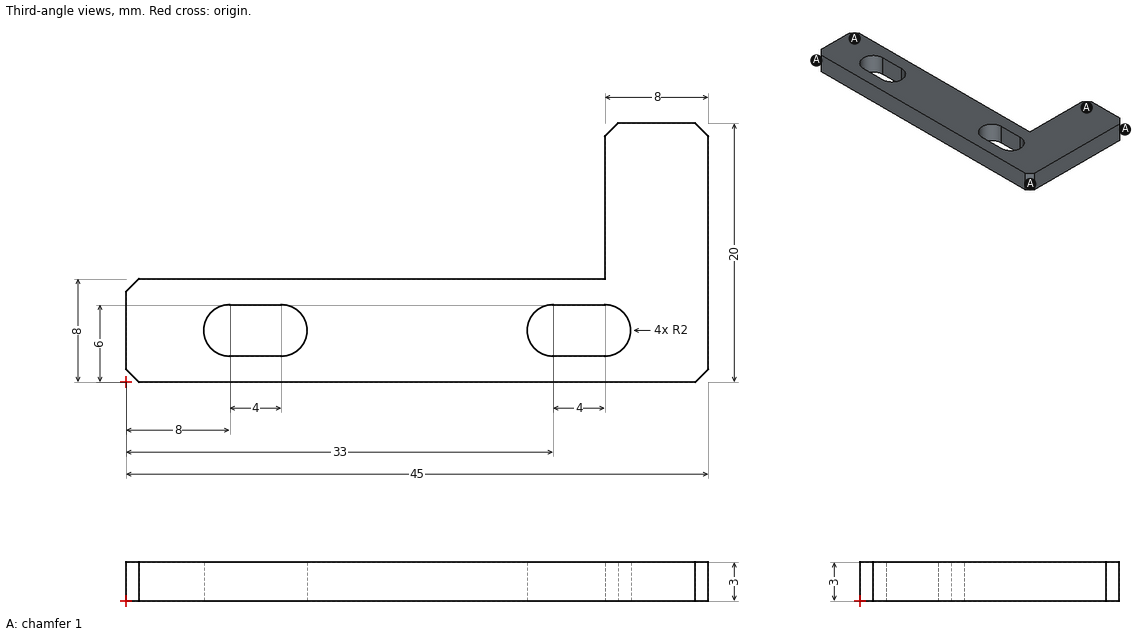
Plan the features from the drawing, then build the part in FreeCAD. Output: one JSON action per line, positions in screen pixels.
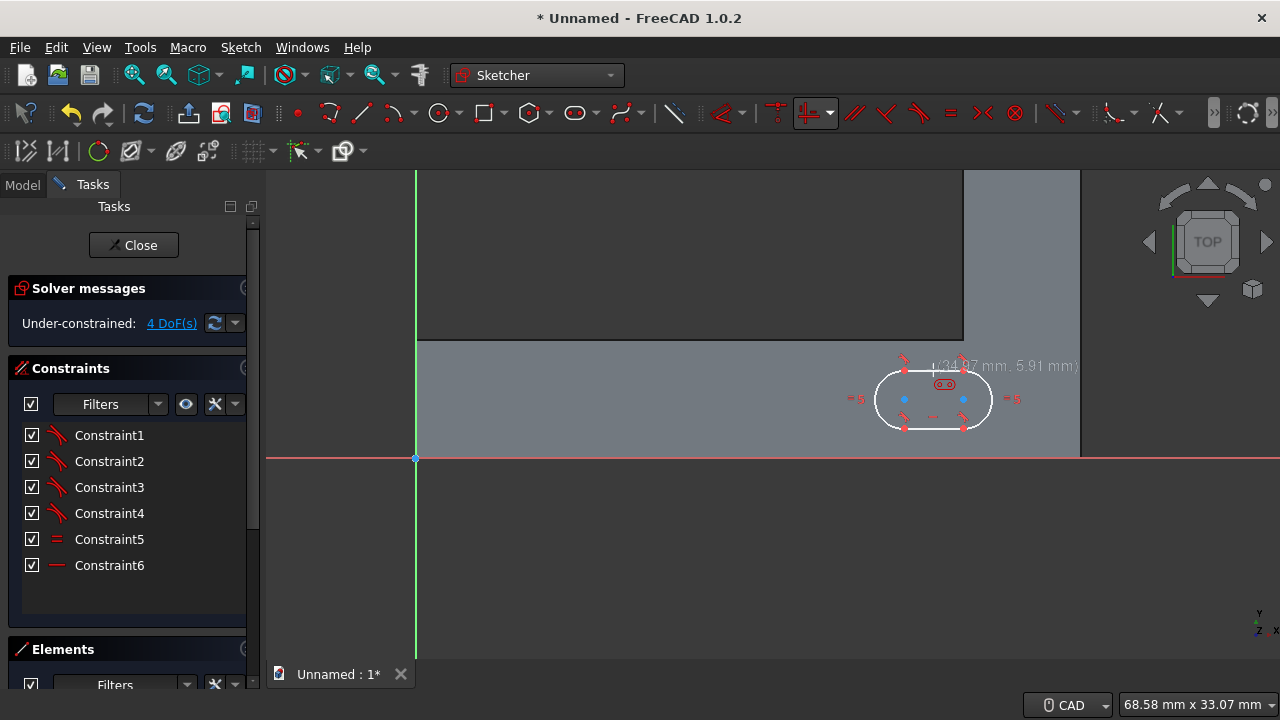
{"action": "left_click", "coordinate": [534, 399]}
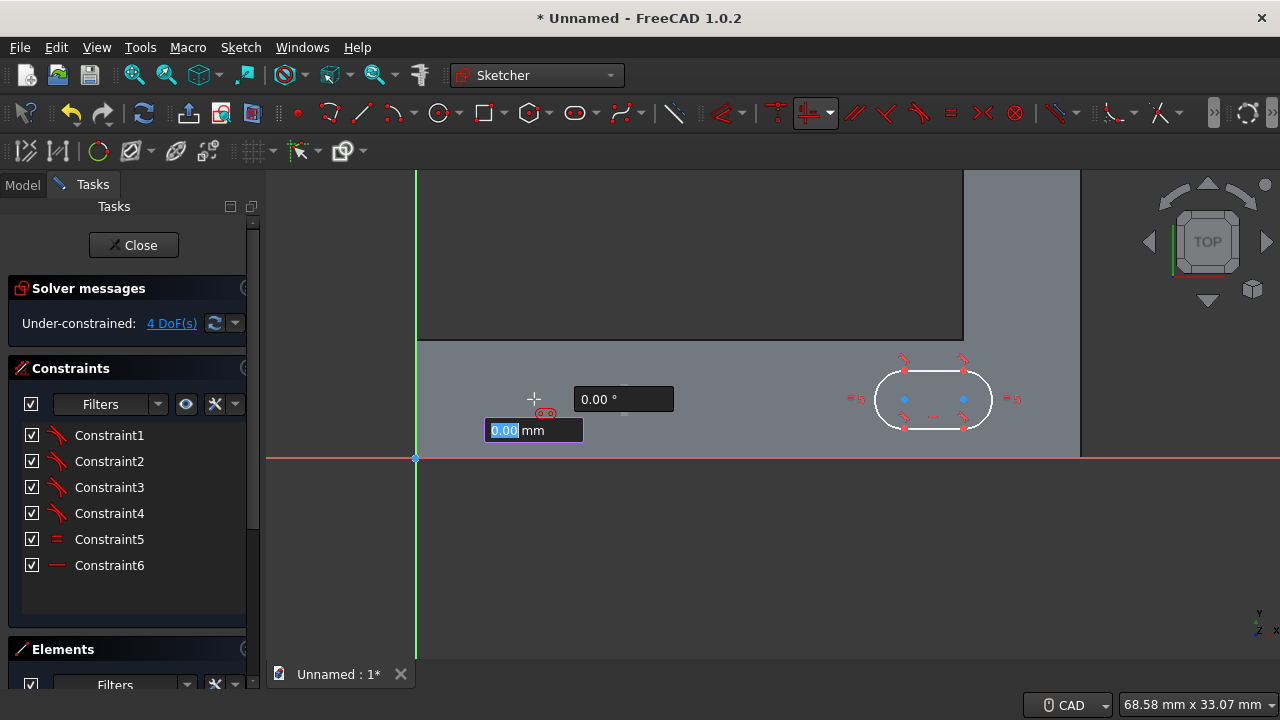
{"action": "left_click", "coordinate": [593, 399]}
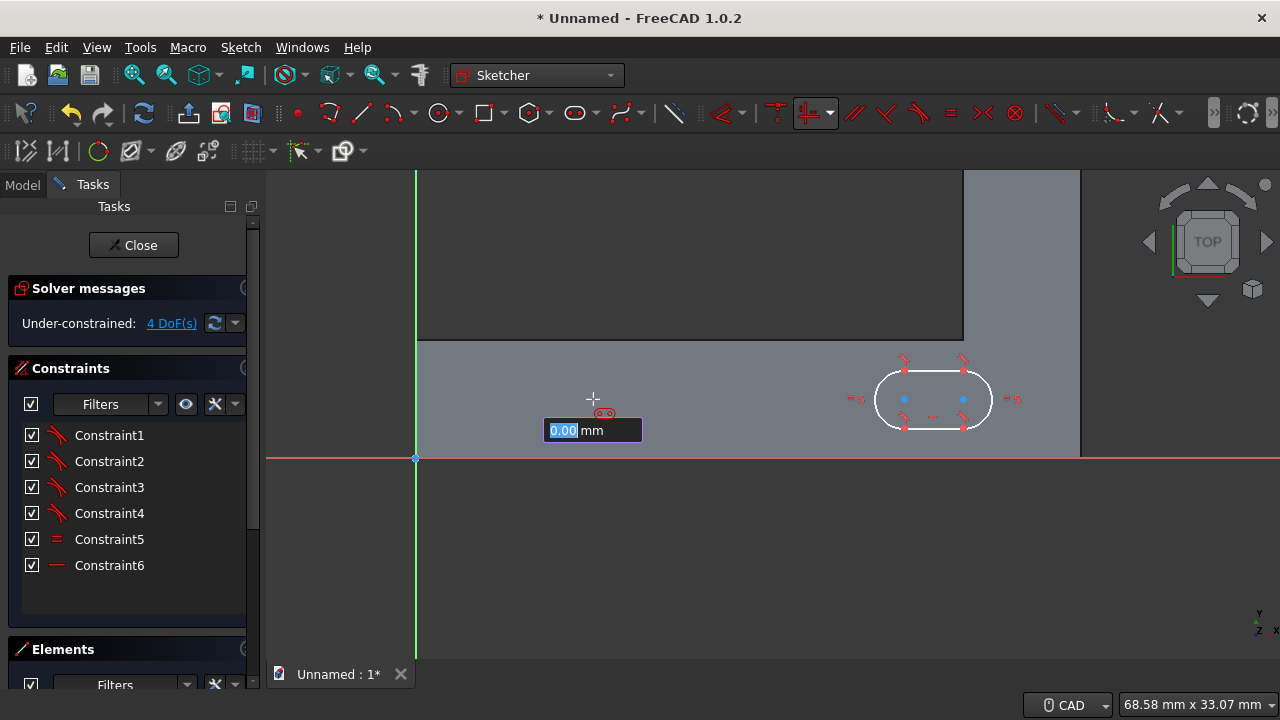
{"action": "left_click", "coordinate": [564, 370]}
{"action": "key", "text": "Escape"}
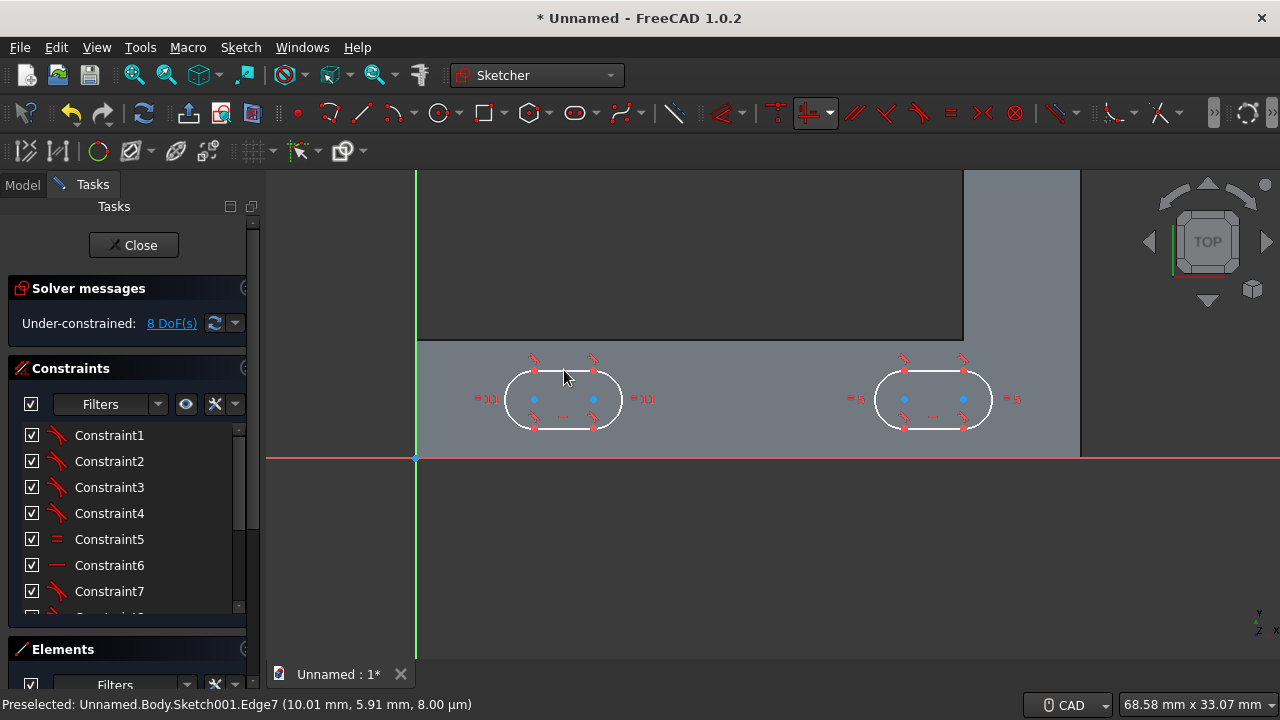
{"action": "left_click", "coordinate": [881, 383]}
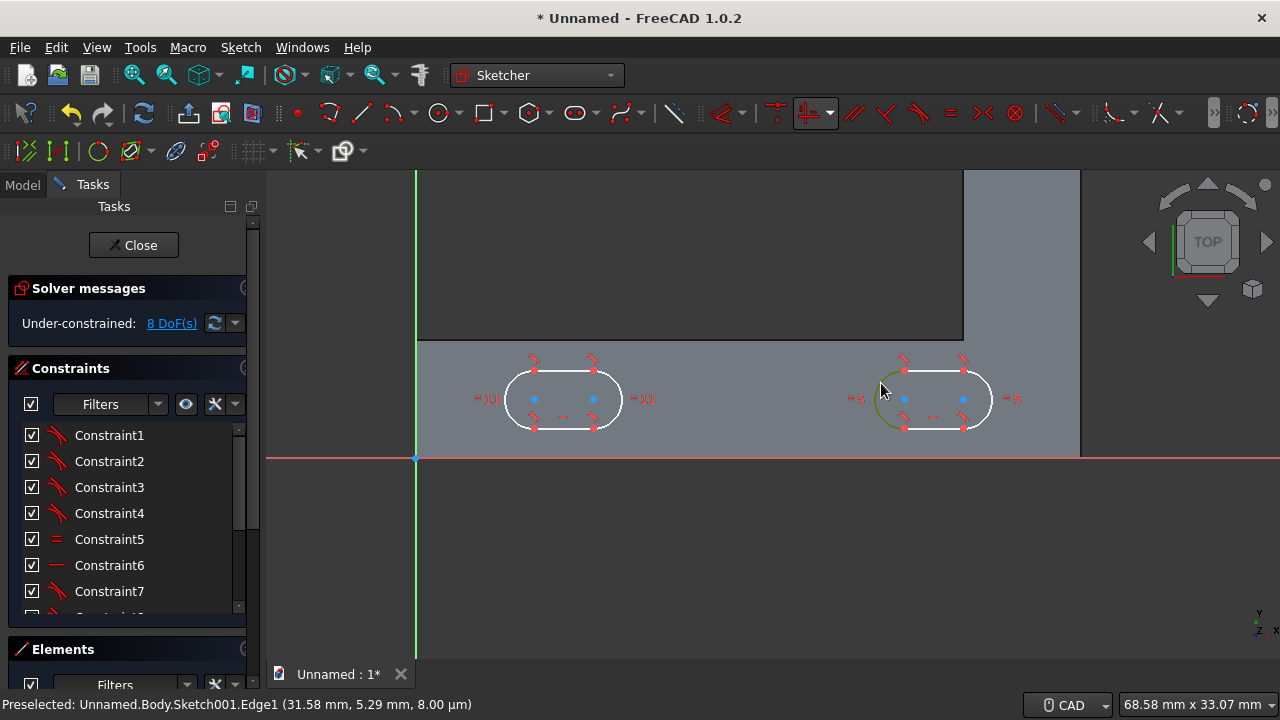
{"action": "left_click", "coordinate": [511, 383]}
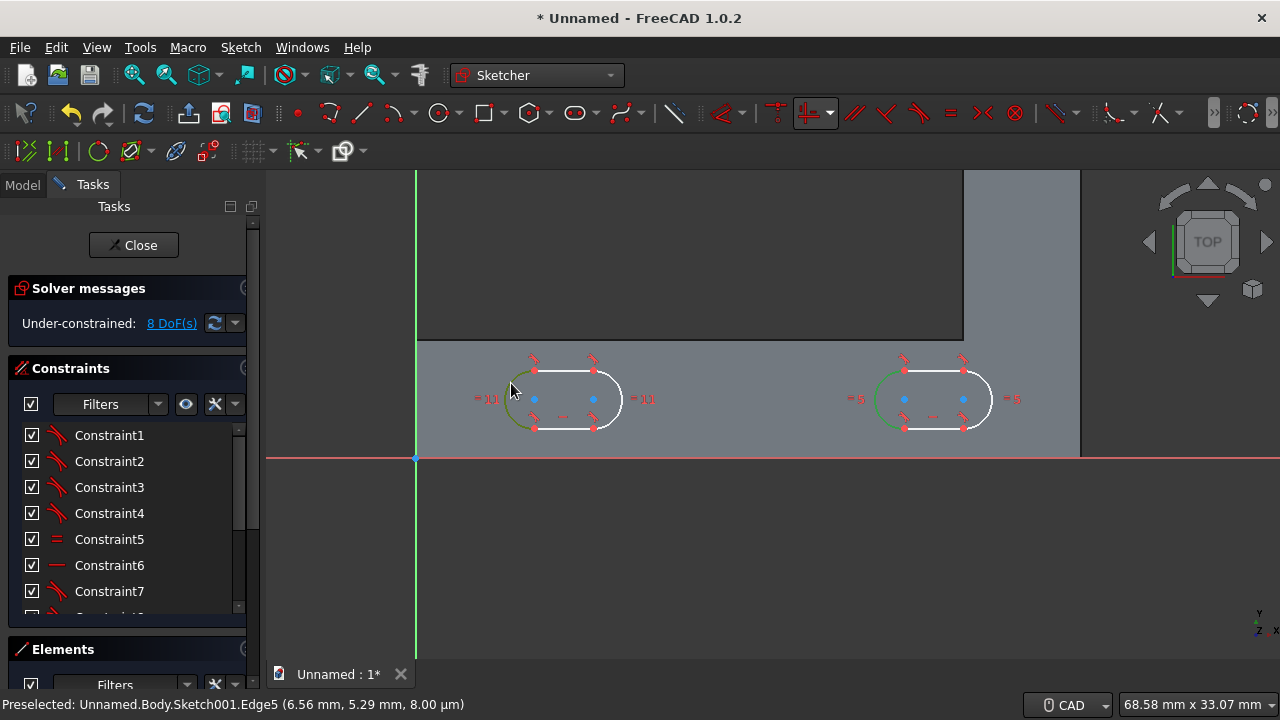
{"action": "left_click", "coordinate": [952, 114]}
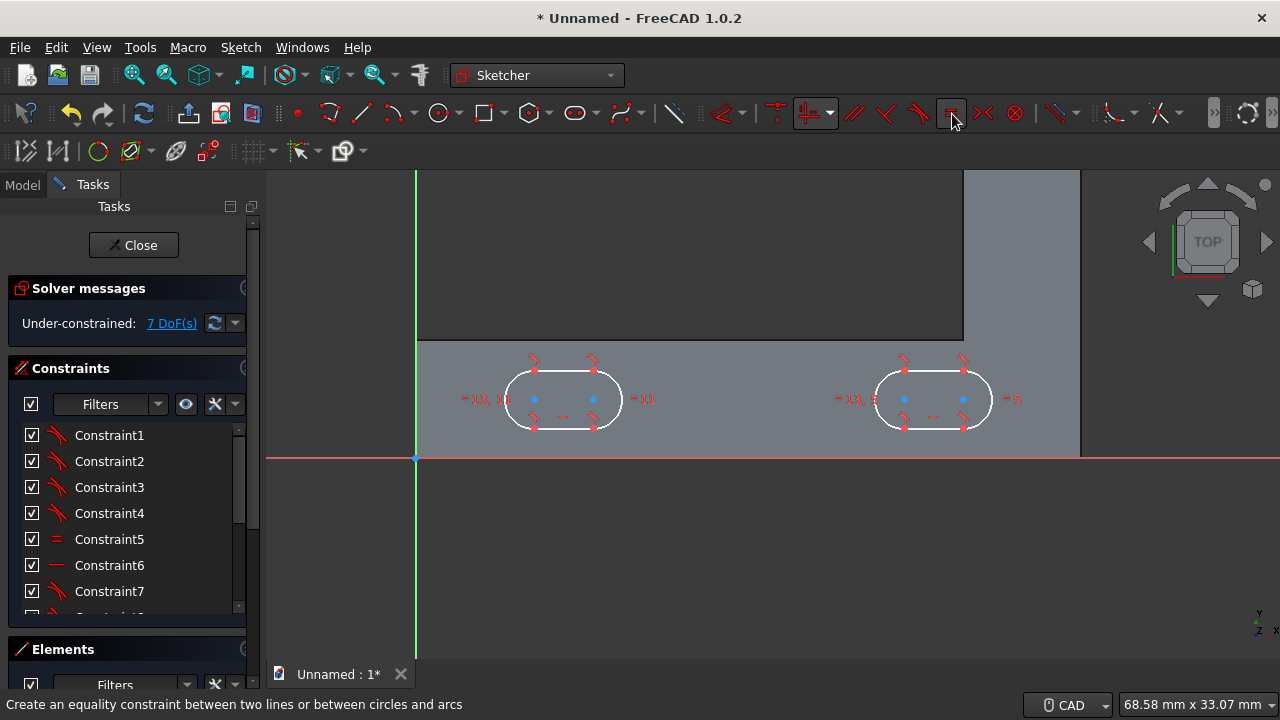
{"action": "left_click", "coordinate": [722, 114]}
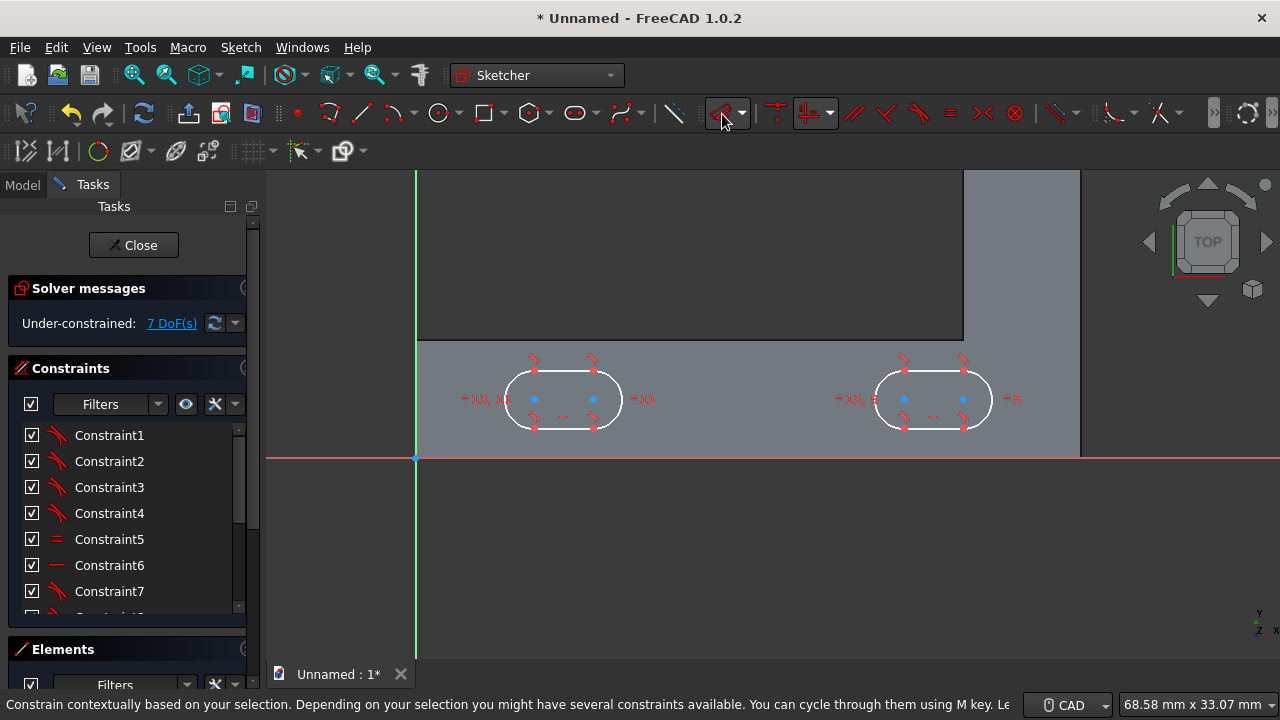
{"action": "scroll", "coordinate": [881, 383], "scroll_direction": "up", "scroll_amount": 2}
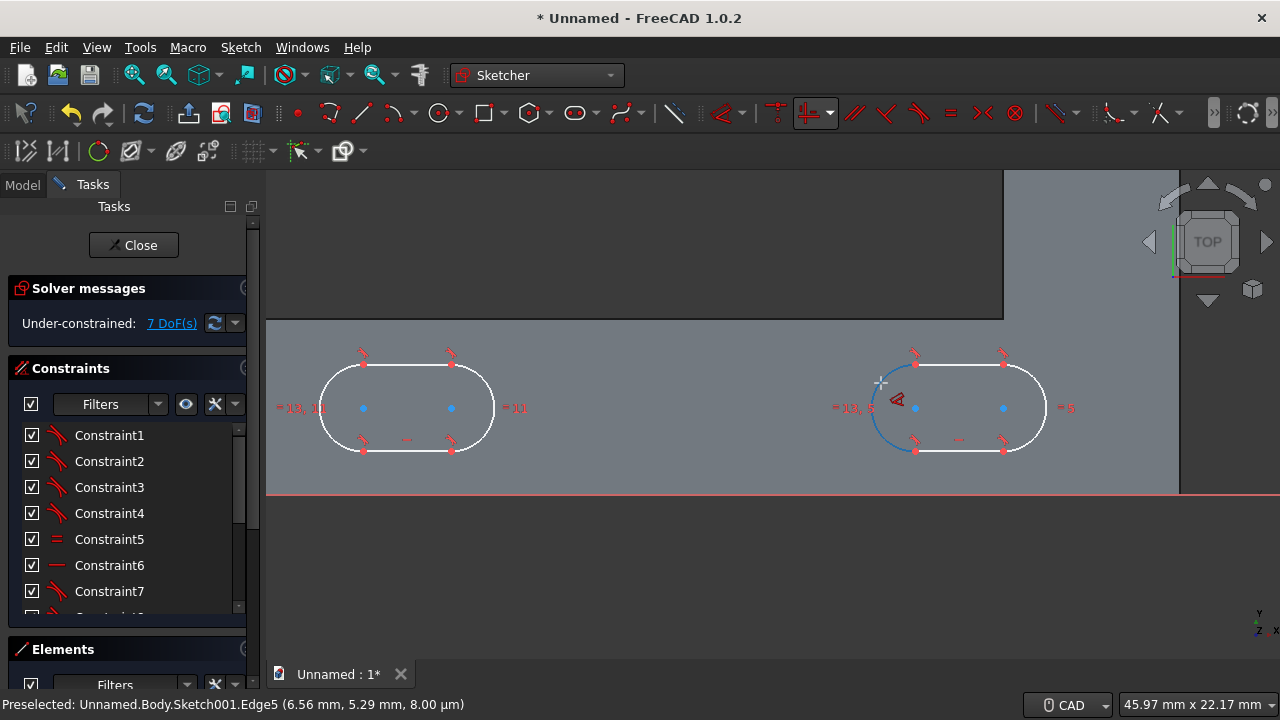
{"action": "left_click", "coordinate": [880, 383]}
{"action": "left_click", "coordinate": [854, 364]}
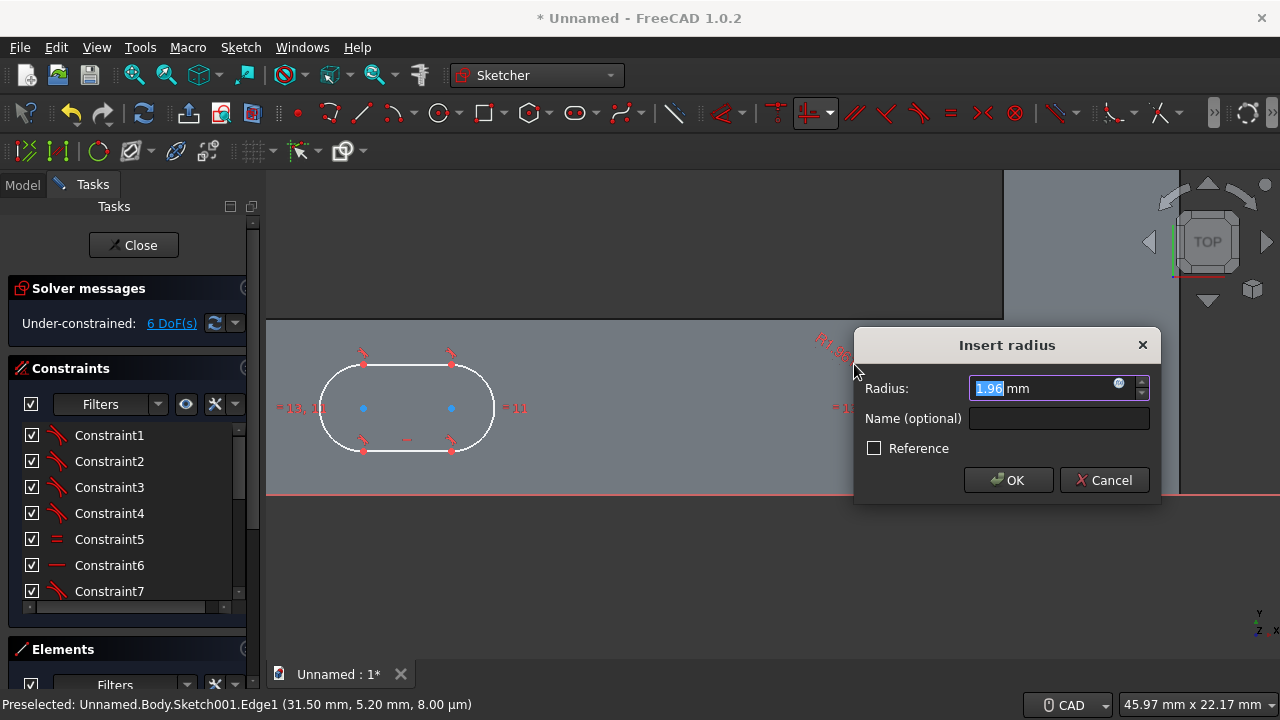
{"action": "type", "text": "2"}
{"action": "key", "text": "Return"}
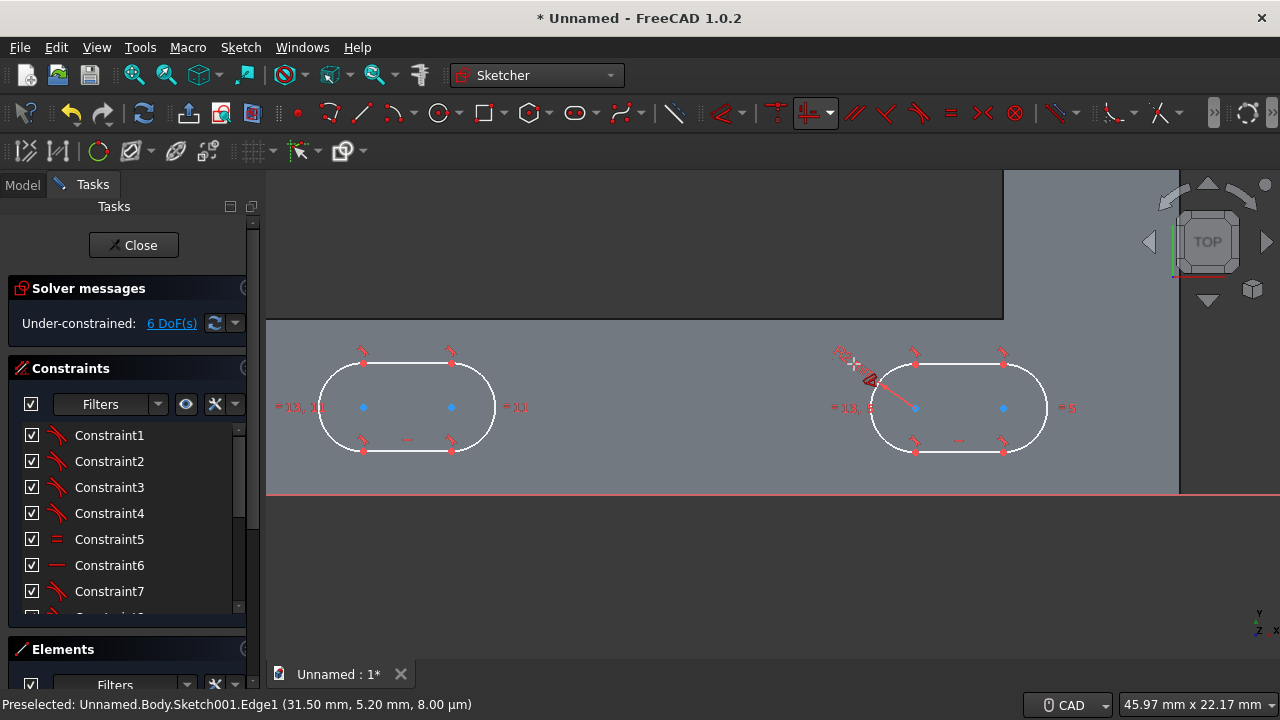
{"action": "left_click", "coordinate": [941, 364]}
{"action": "left_click", "coordinate": [959, 330]}